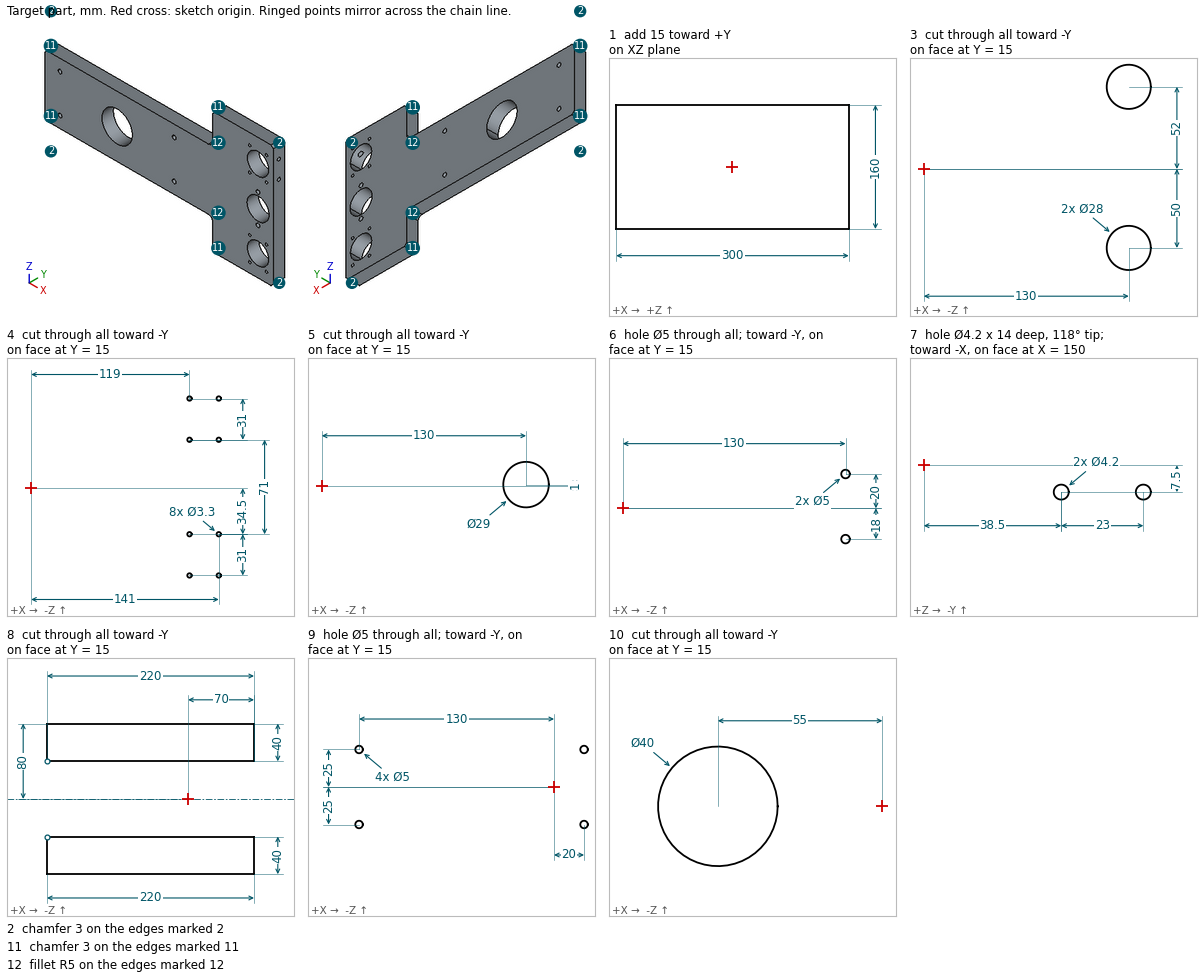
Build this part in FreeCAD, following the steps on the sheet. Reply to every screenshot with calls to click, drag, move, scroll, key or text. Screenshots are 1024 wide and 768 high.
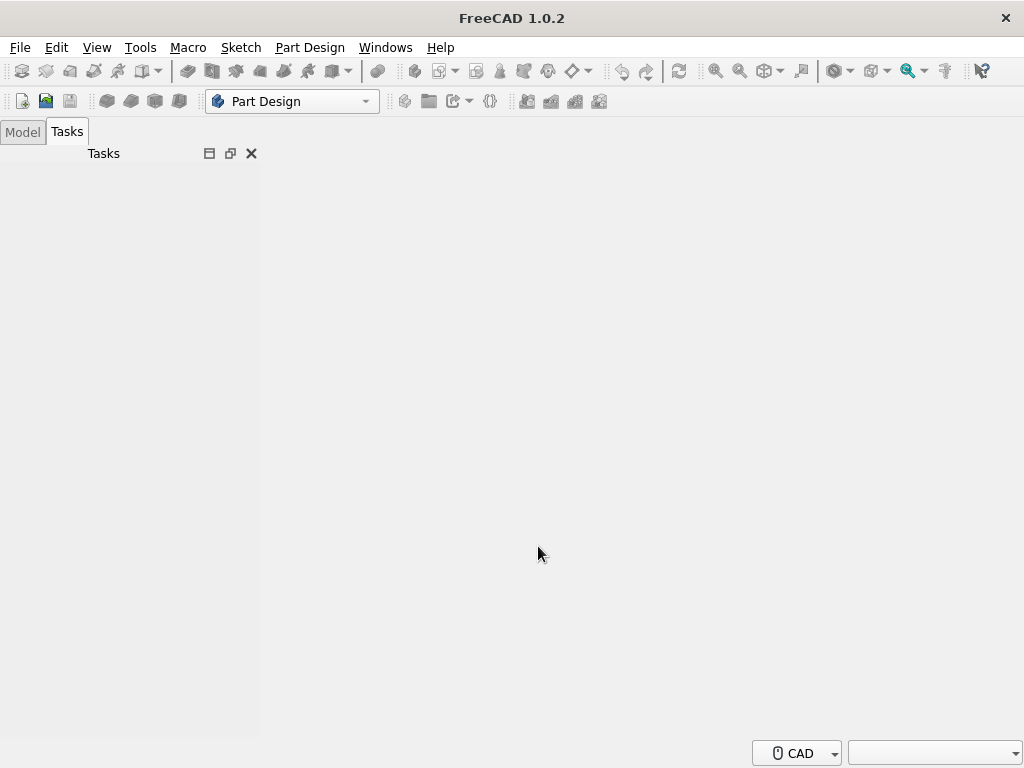
click(22, 102)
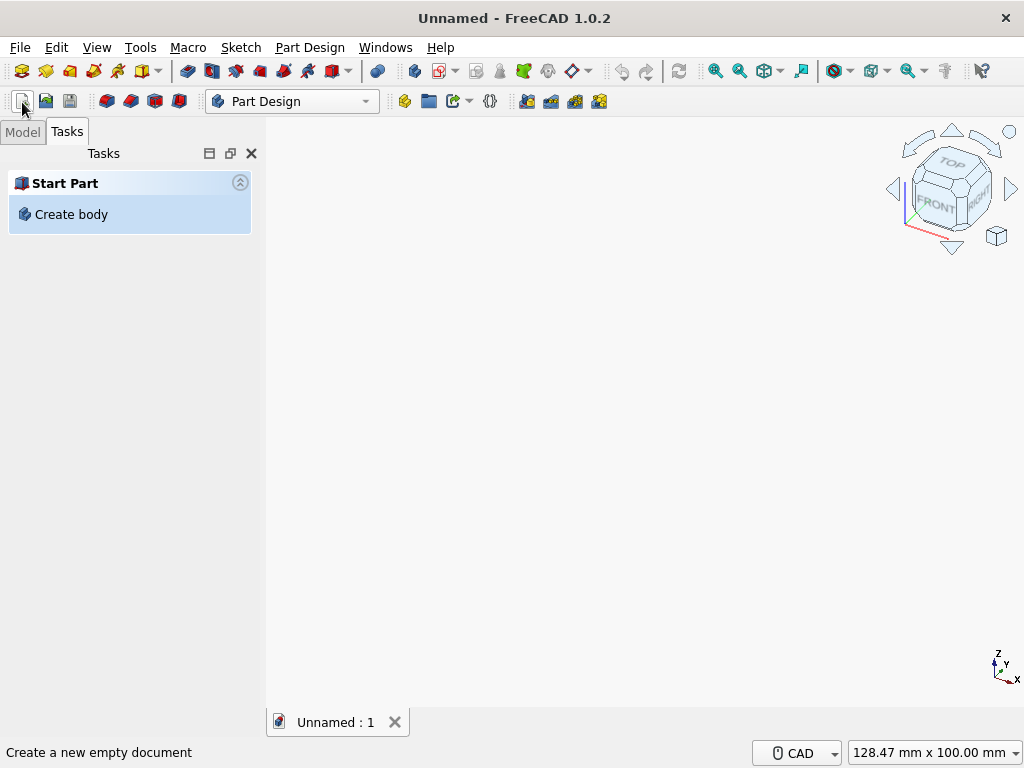
click(440, 72)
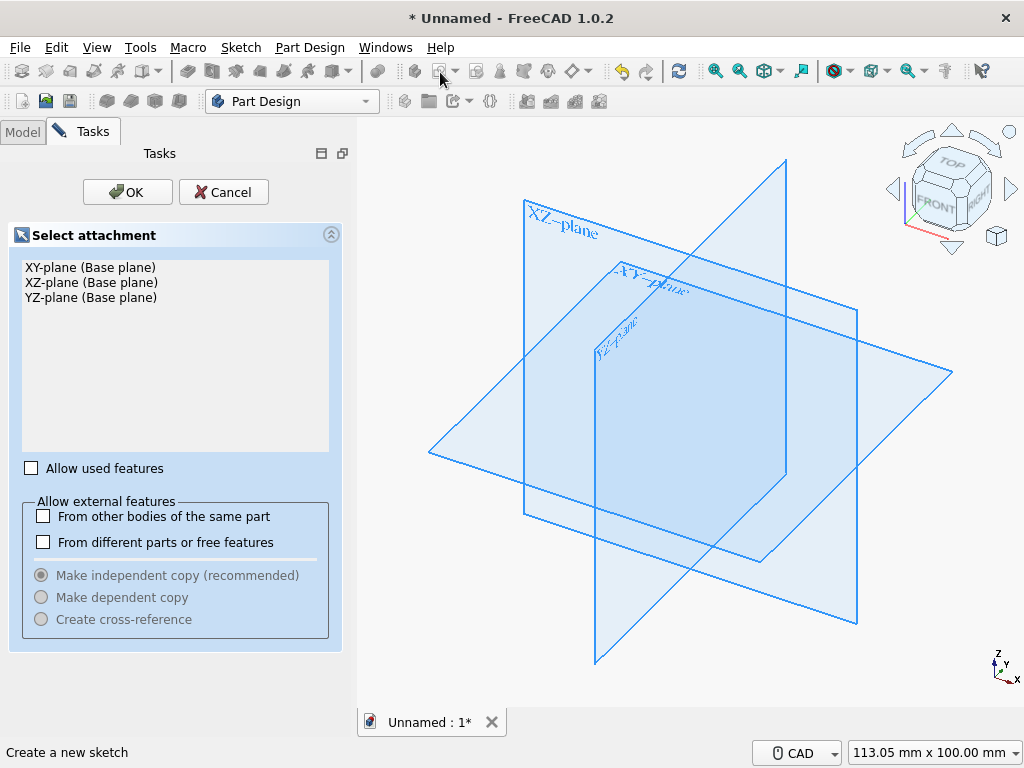
click(82, 282)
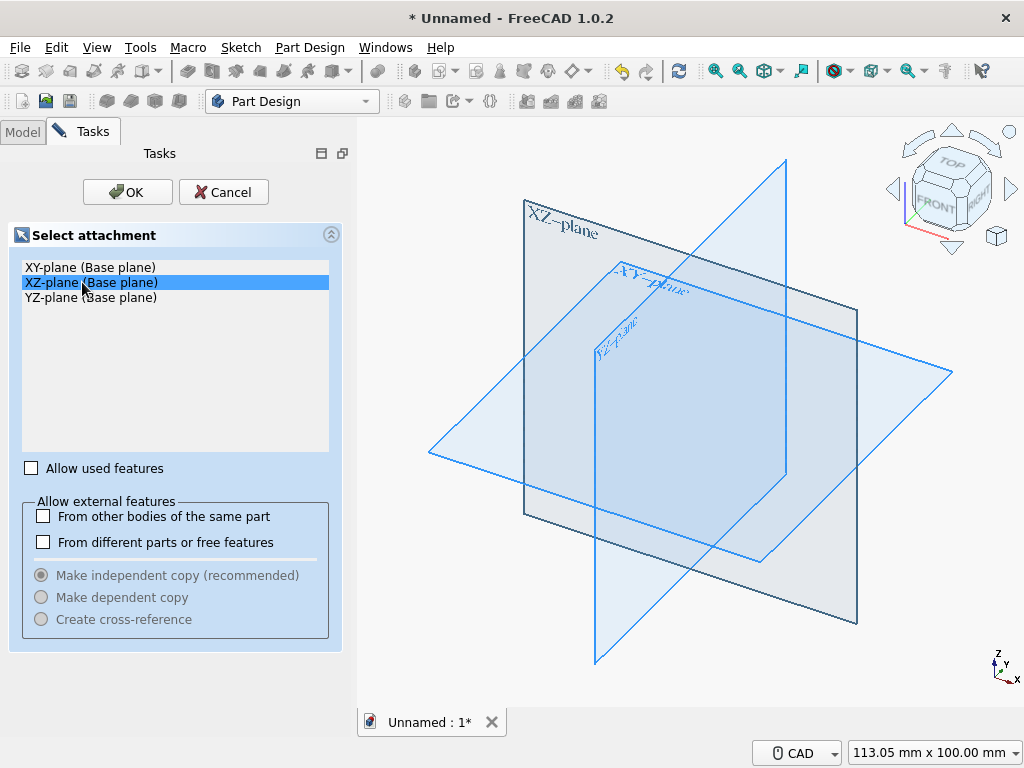
click(128, 192)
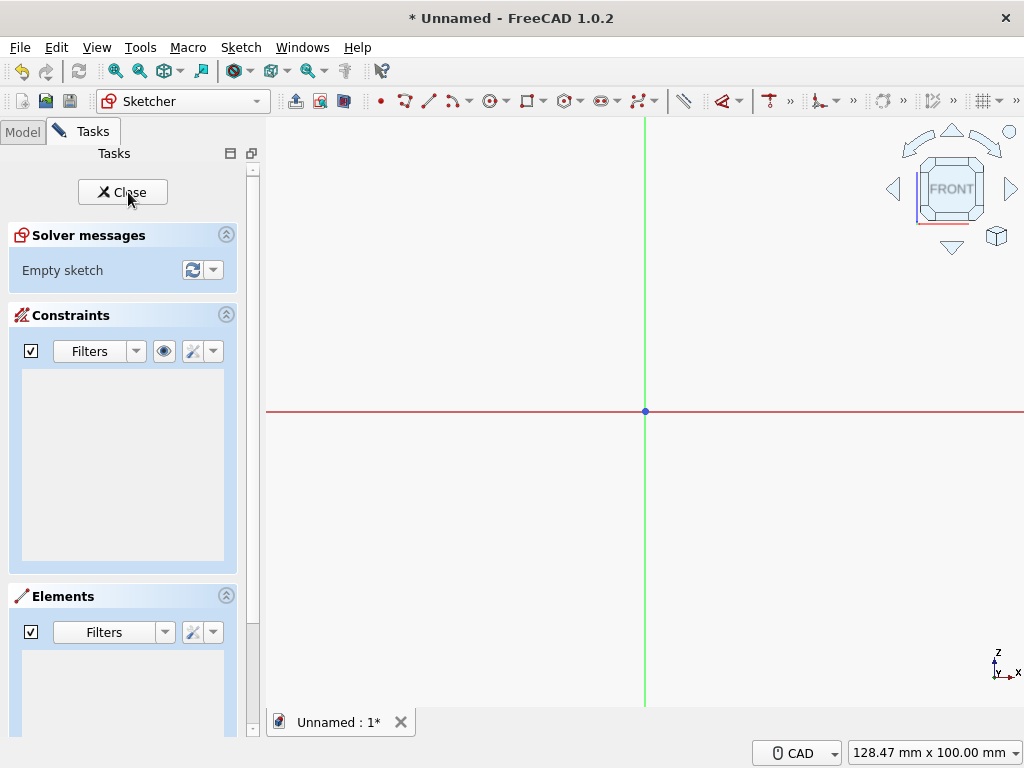
scroll(554, 412, down, 7)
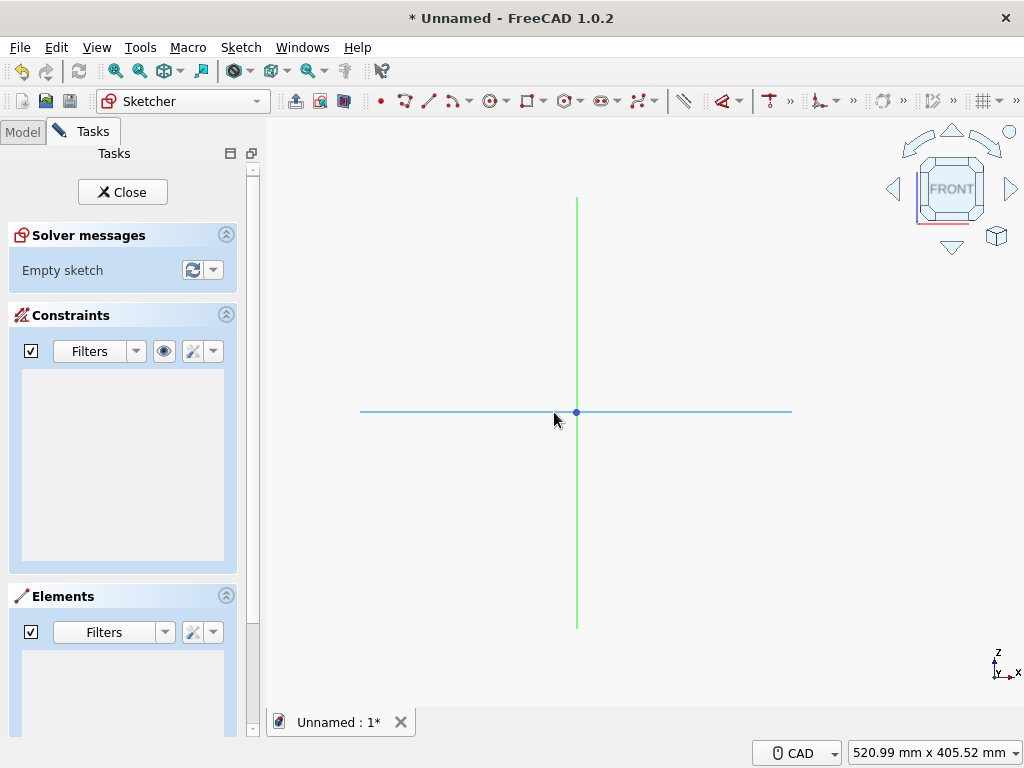
click(546, 102)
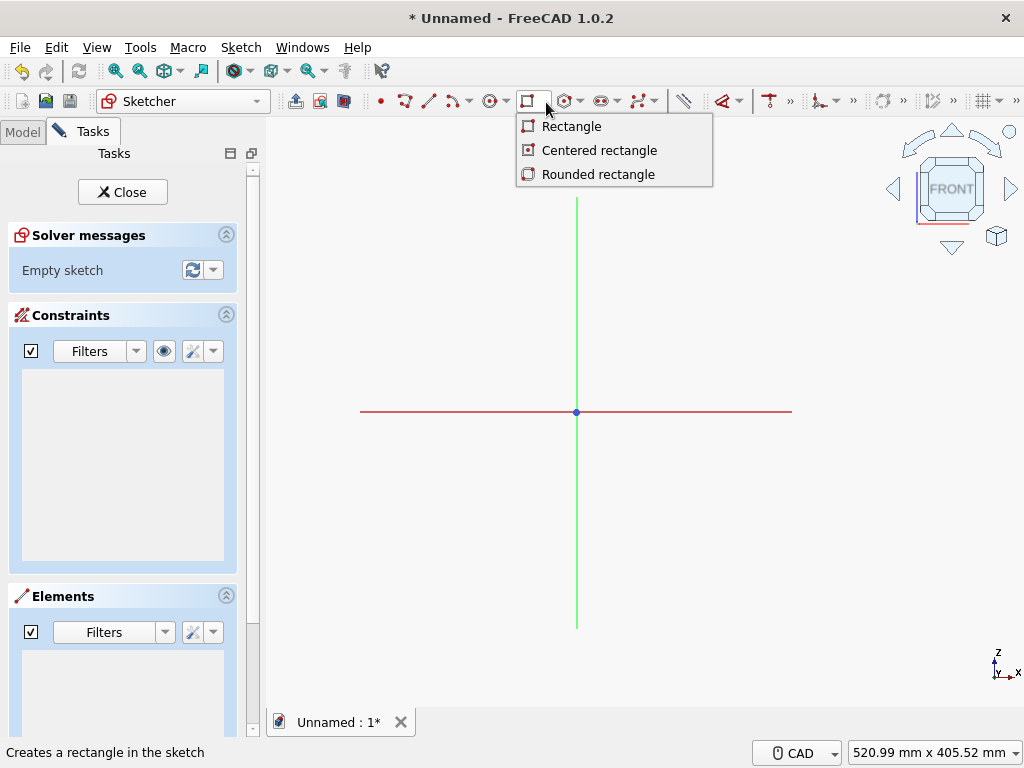
click(614, 150)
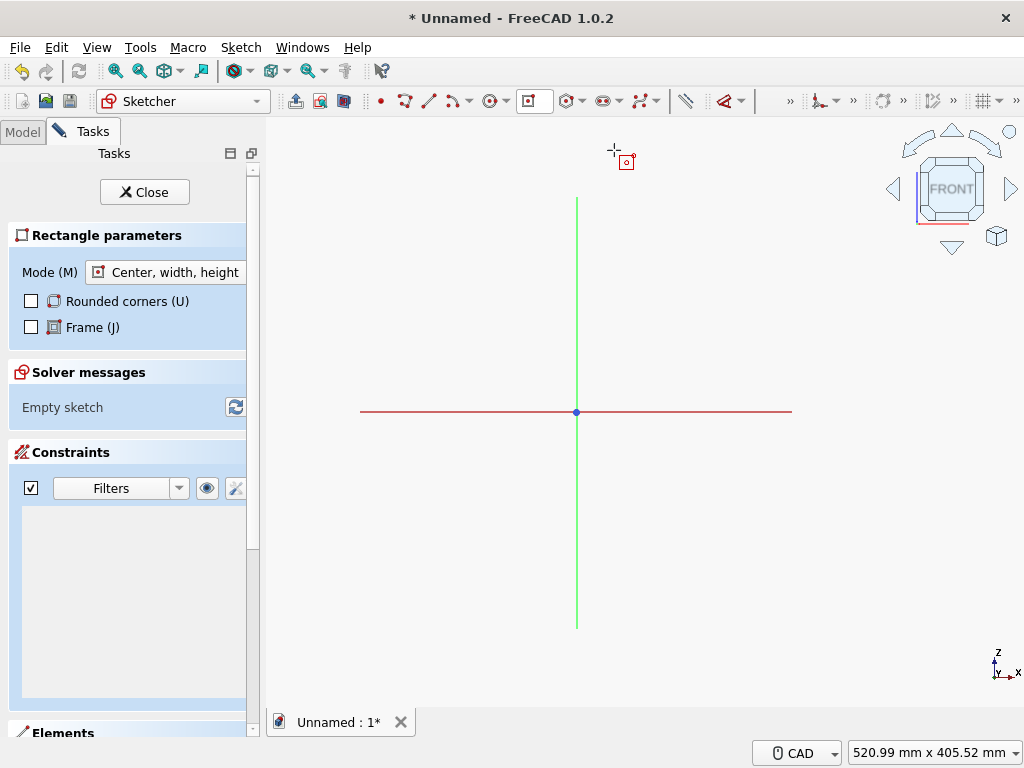
click(577, 412)
move(795, 296)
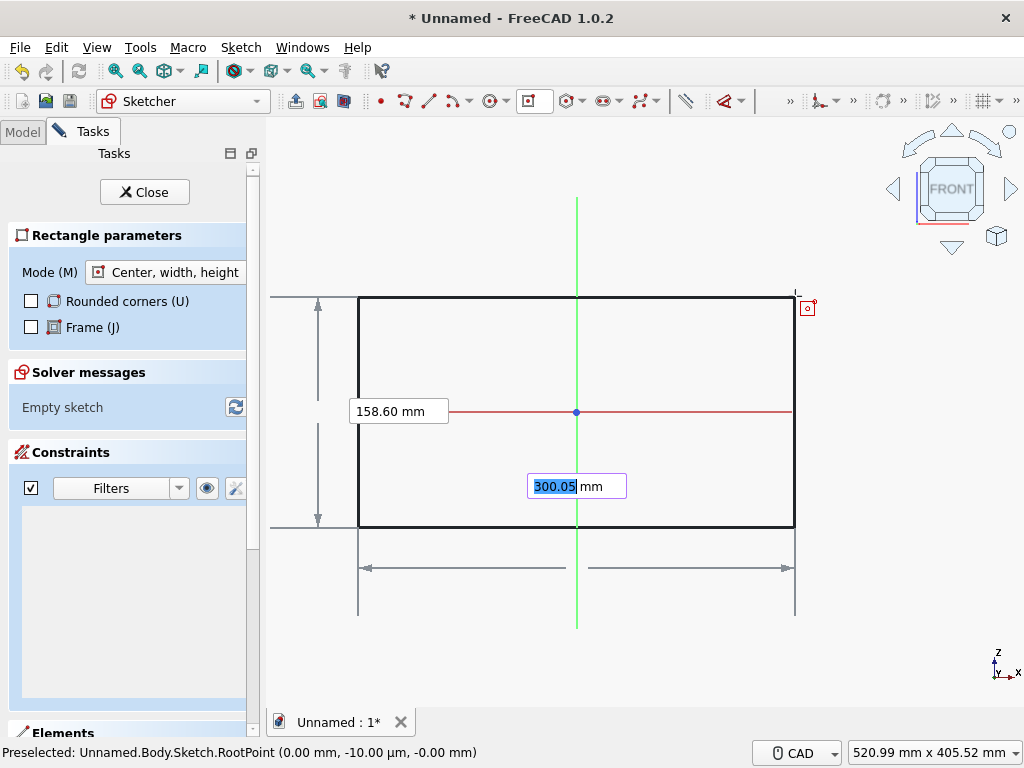
text(300)
key(Tab)
text(160)
key(Return)
key(Escape)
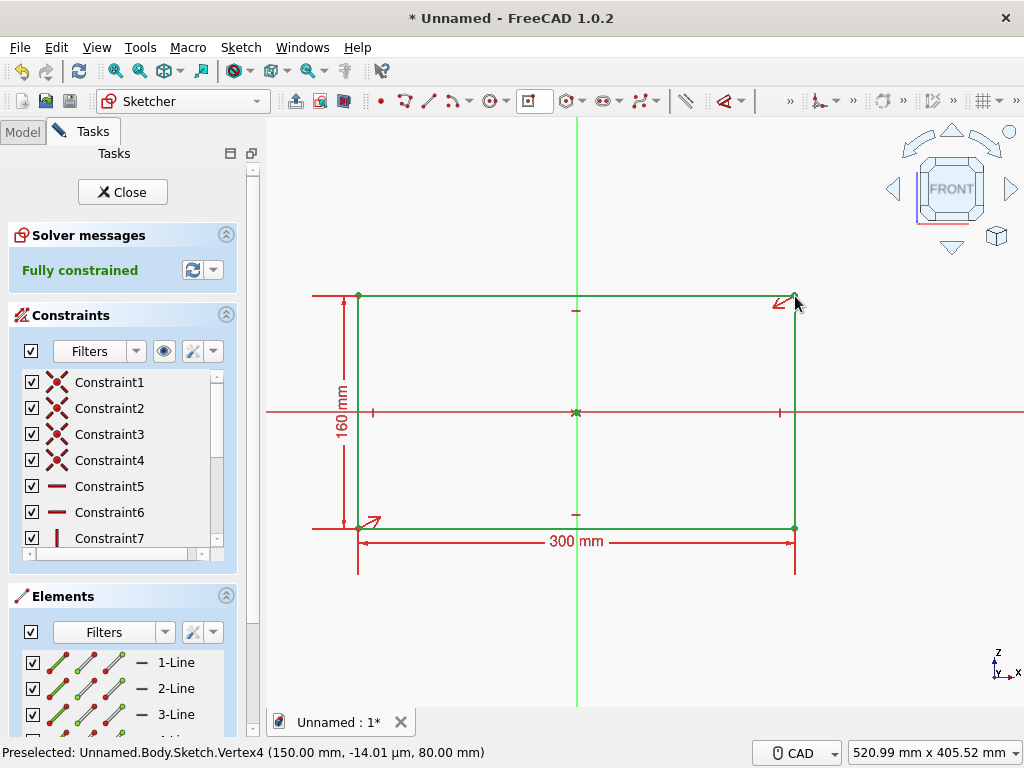
click(123, 192)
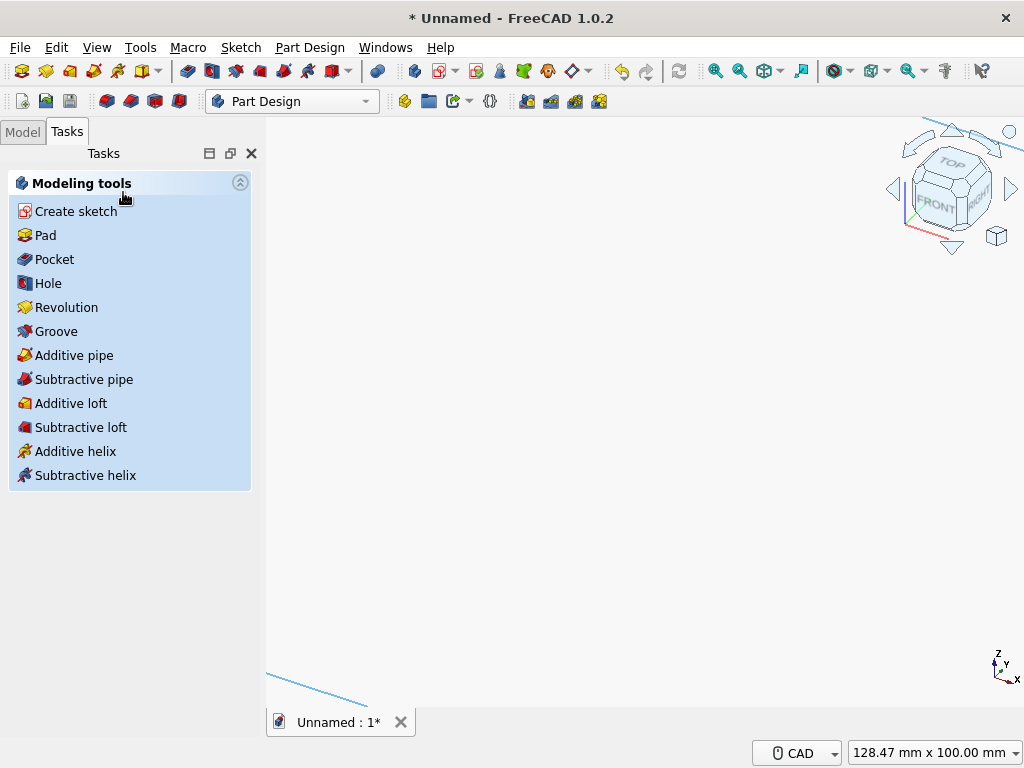
click(22, 72)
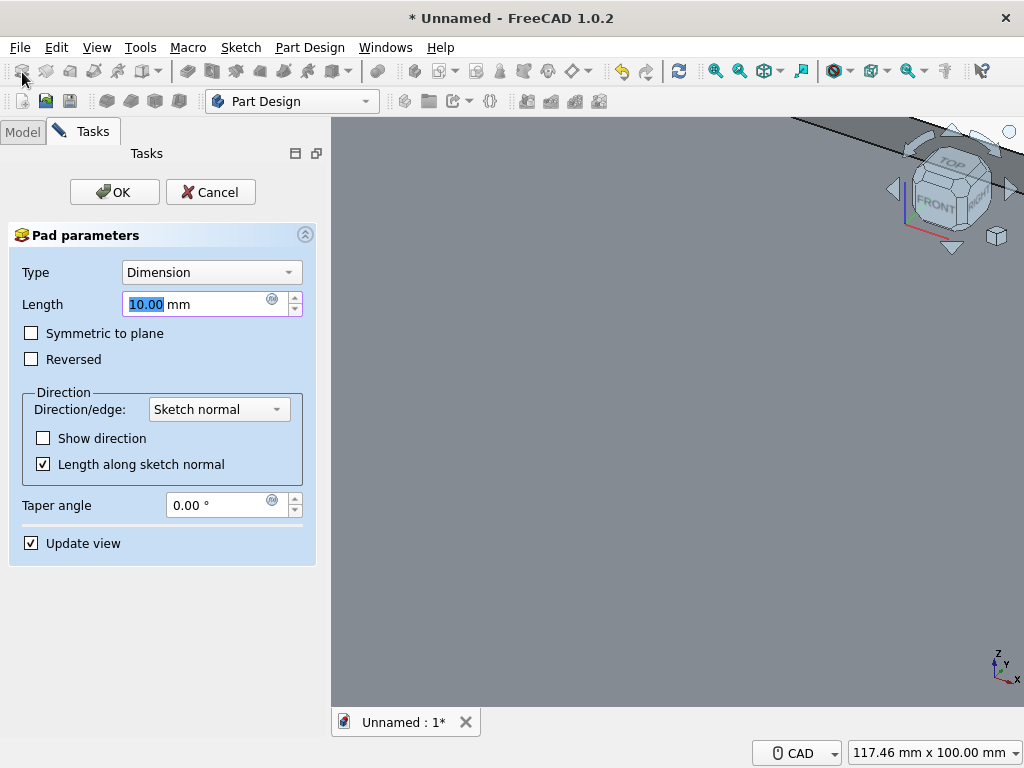
text(15)
key(Tab)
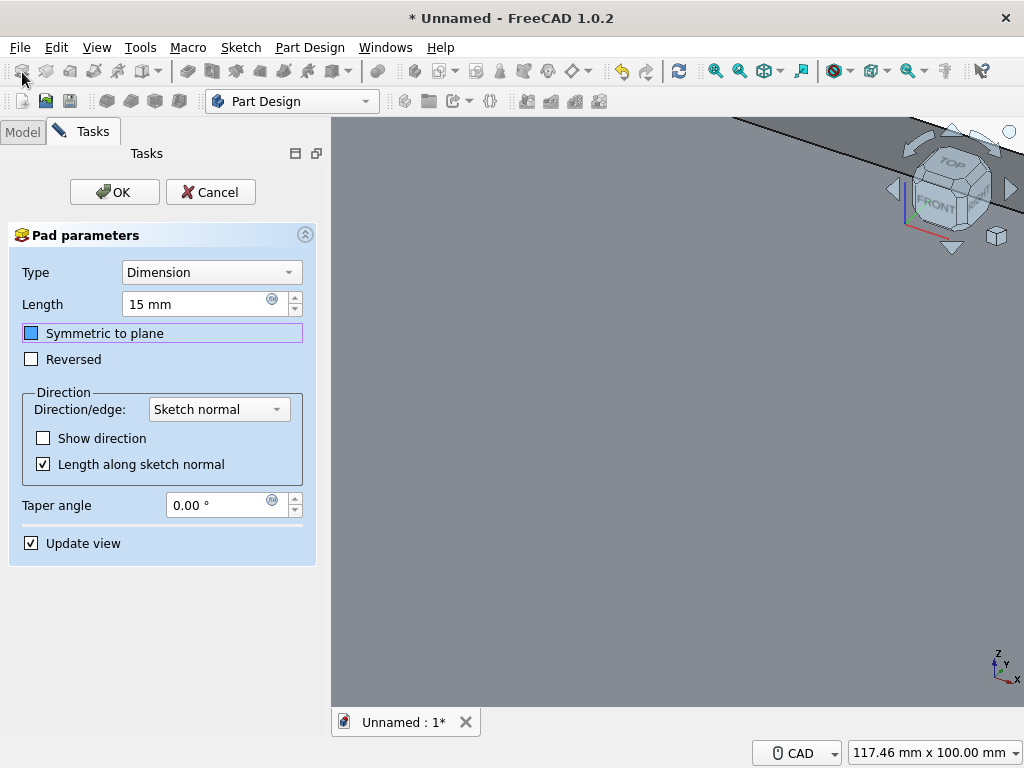
click(30, 359)